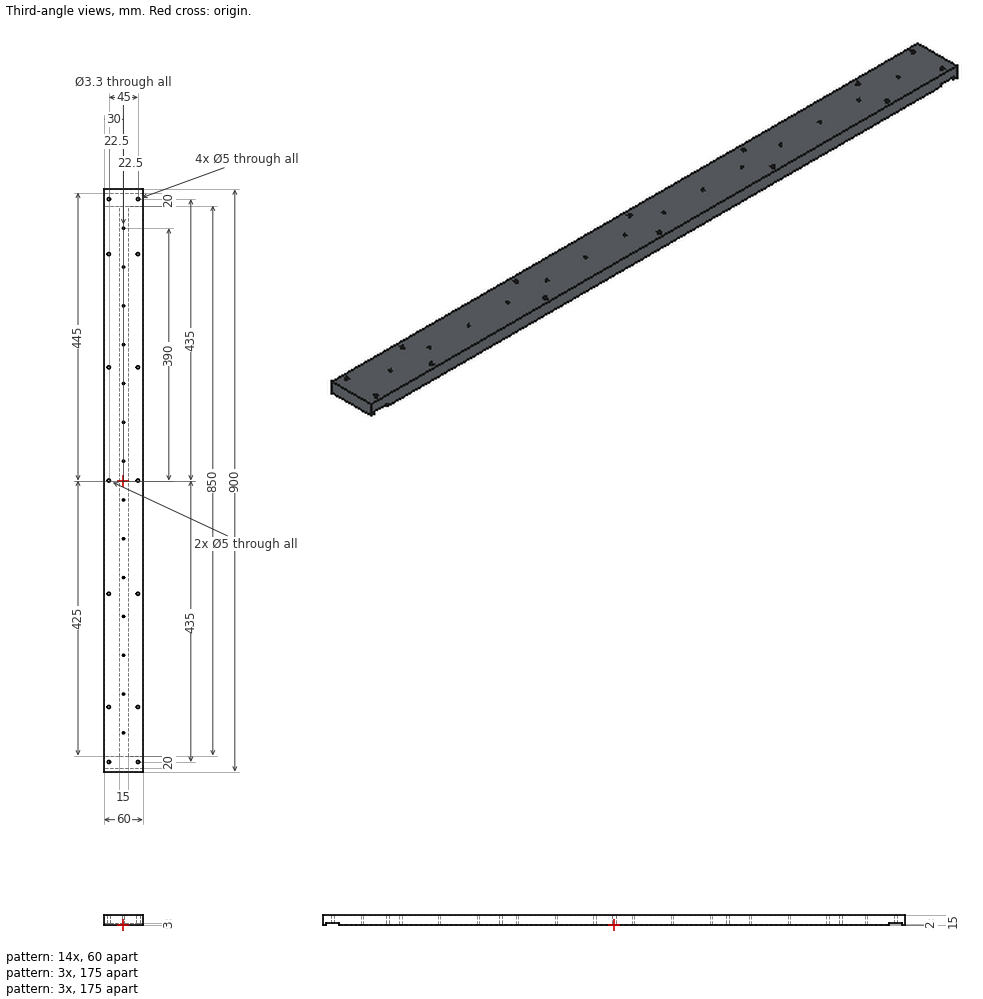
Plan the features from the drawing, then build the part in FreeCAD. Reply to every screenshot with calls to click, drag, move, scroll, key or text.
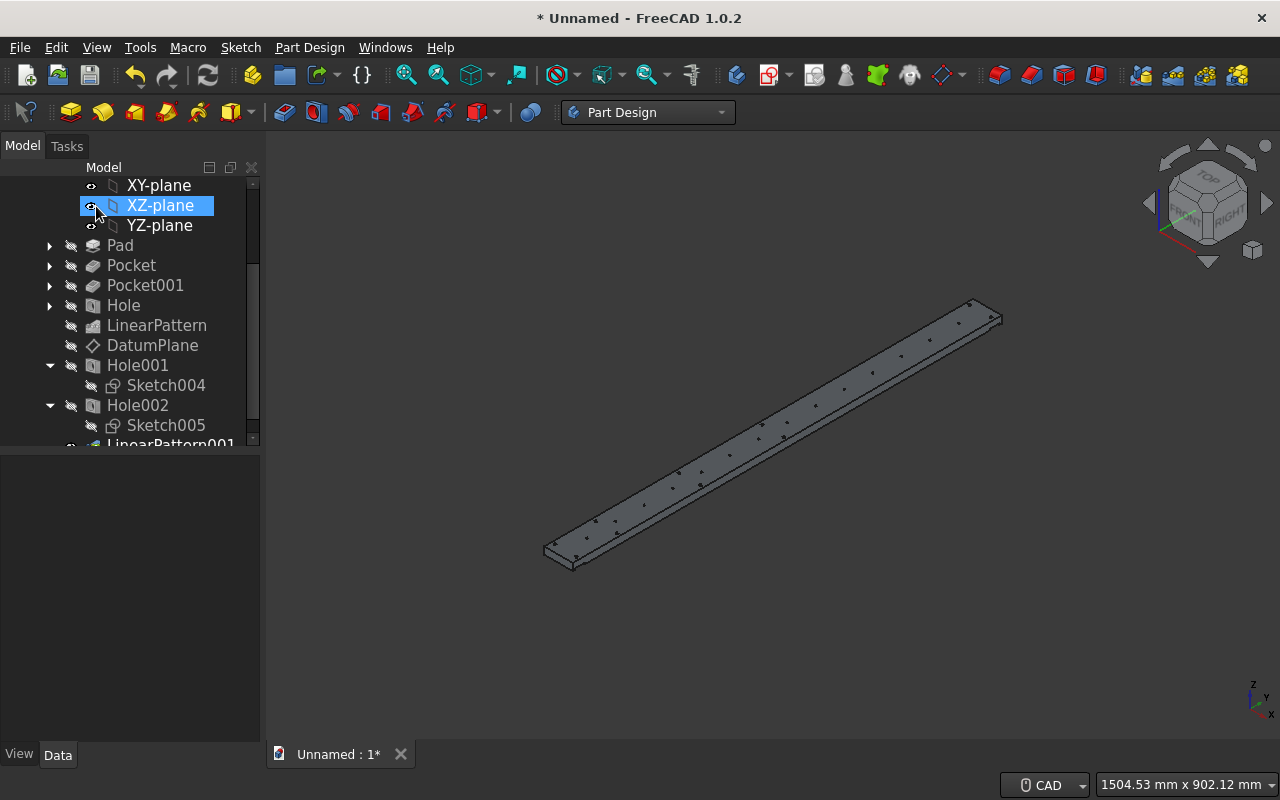
click(116, 406)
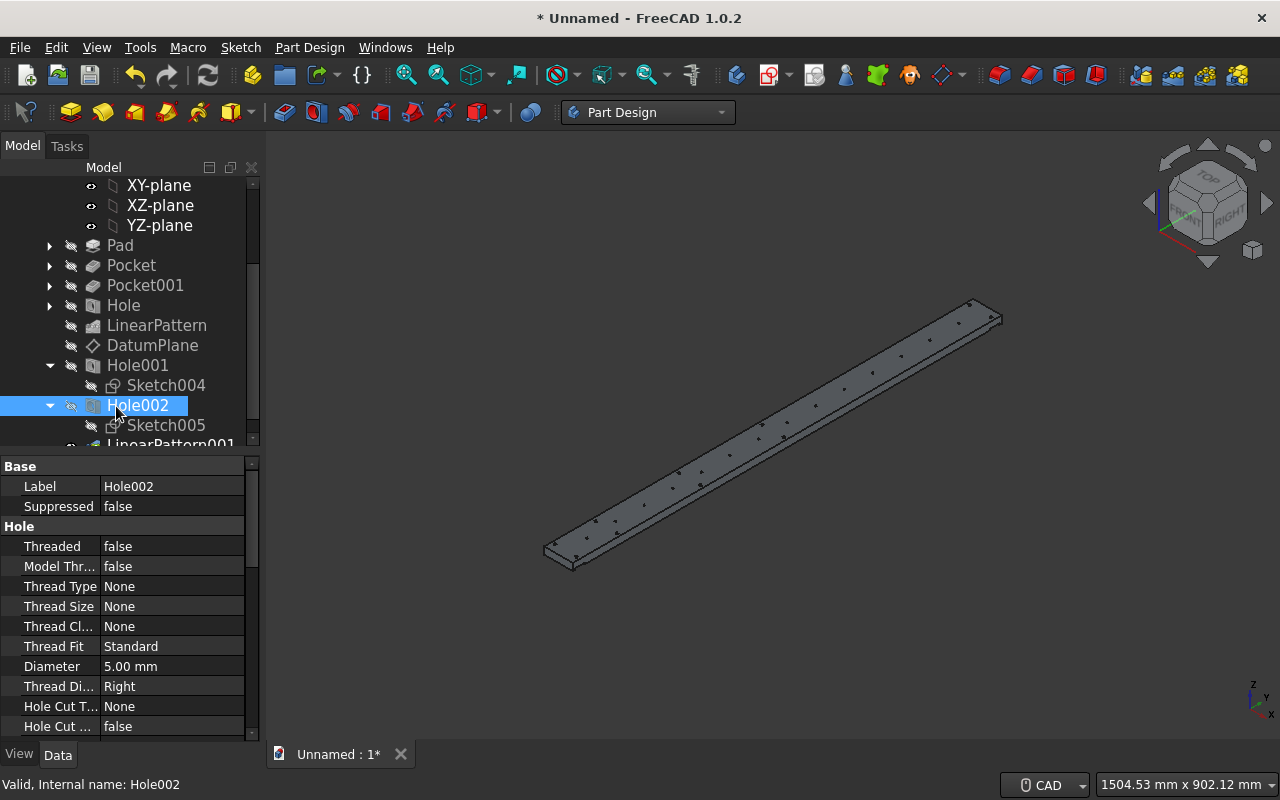
click(1174, 76)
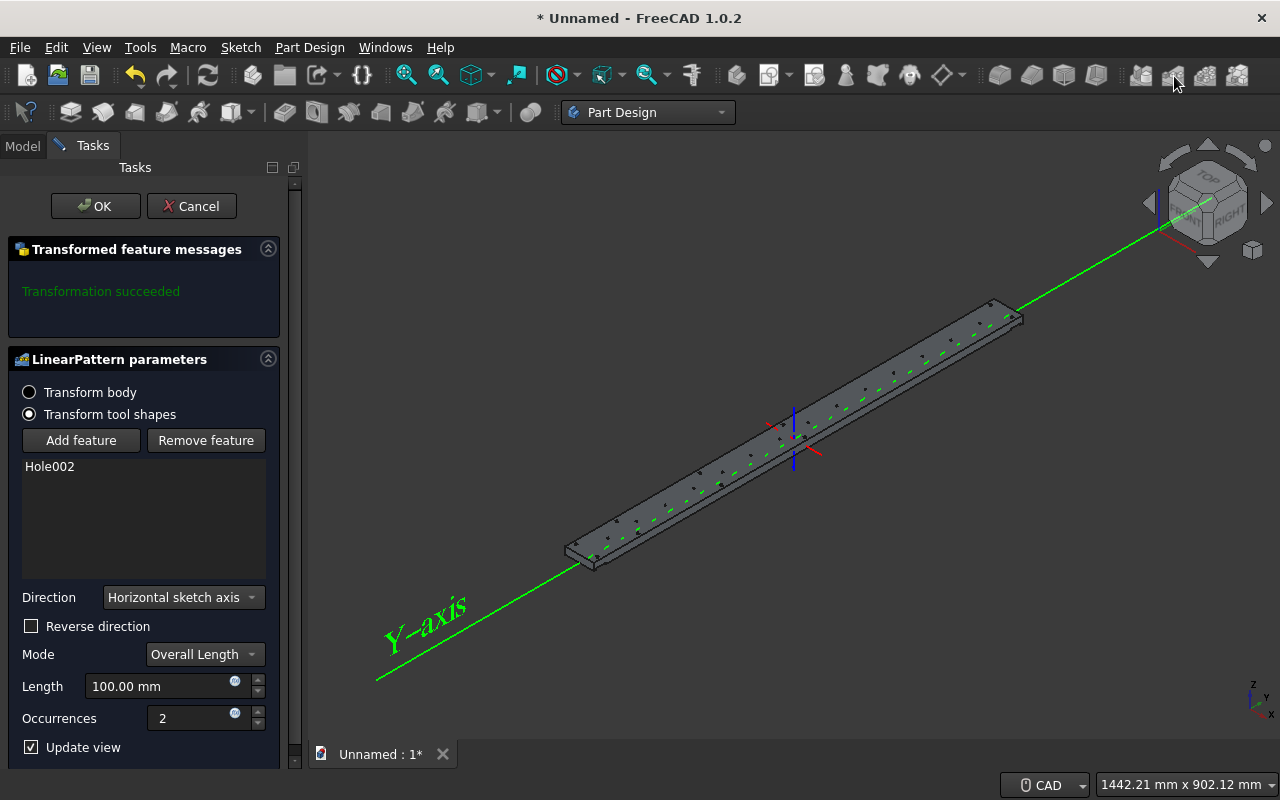
click(184, 598)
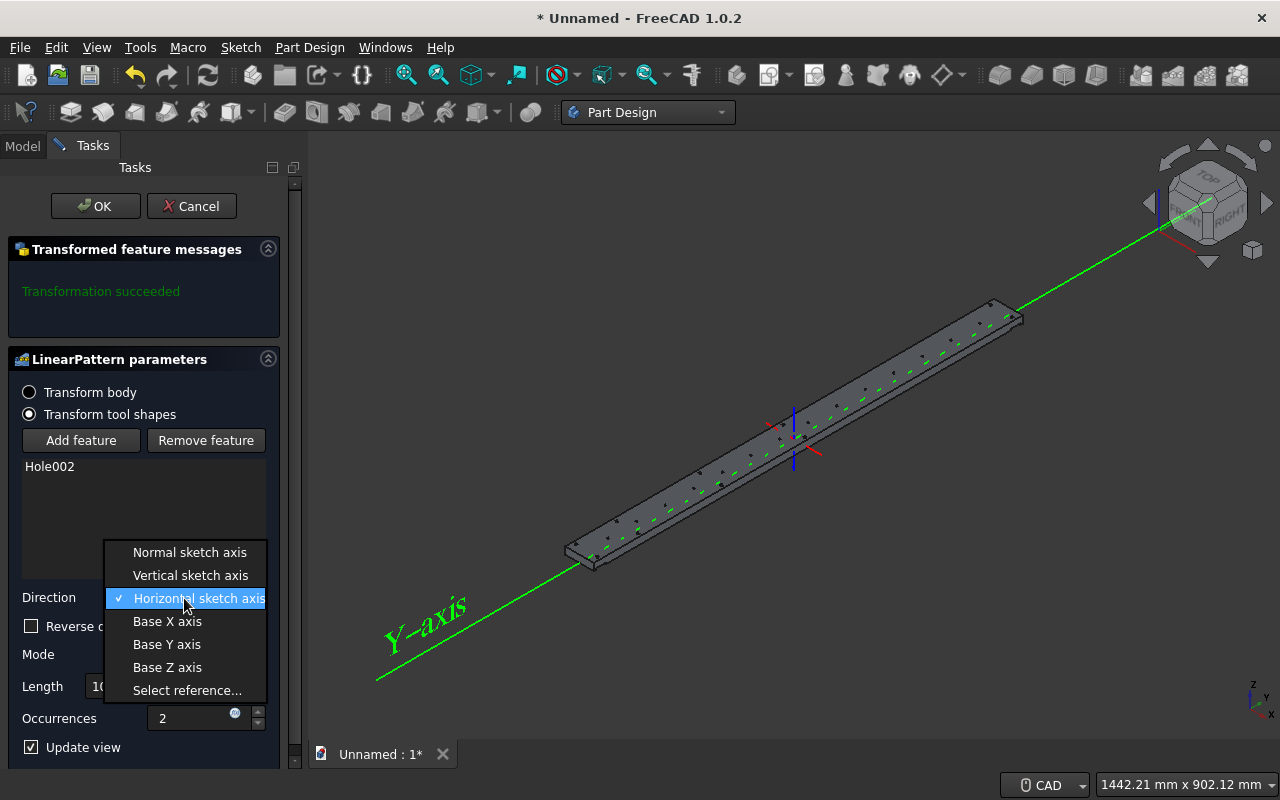
click(184, 644)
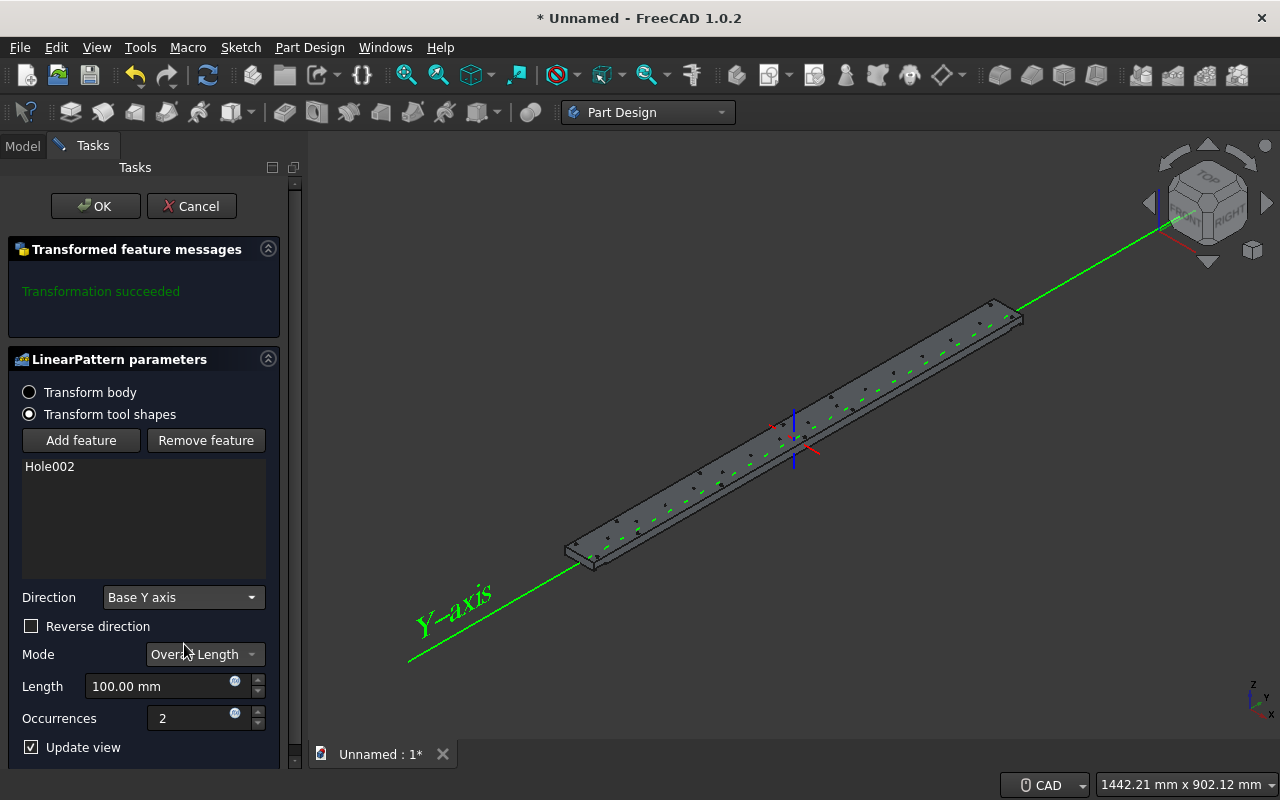
click(206, 654)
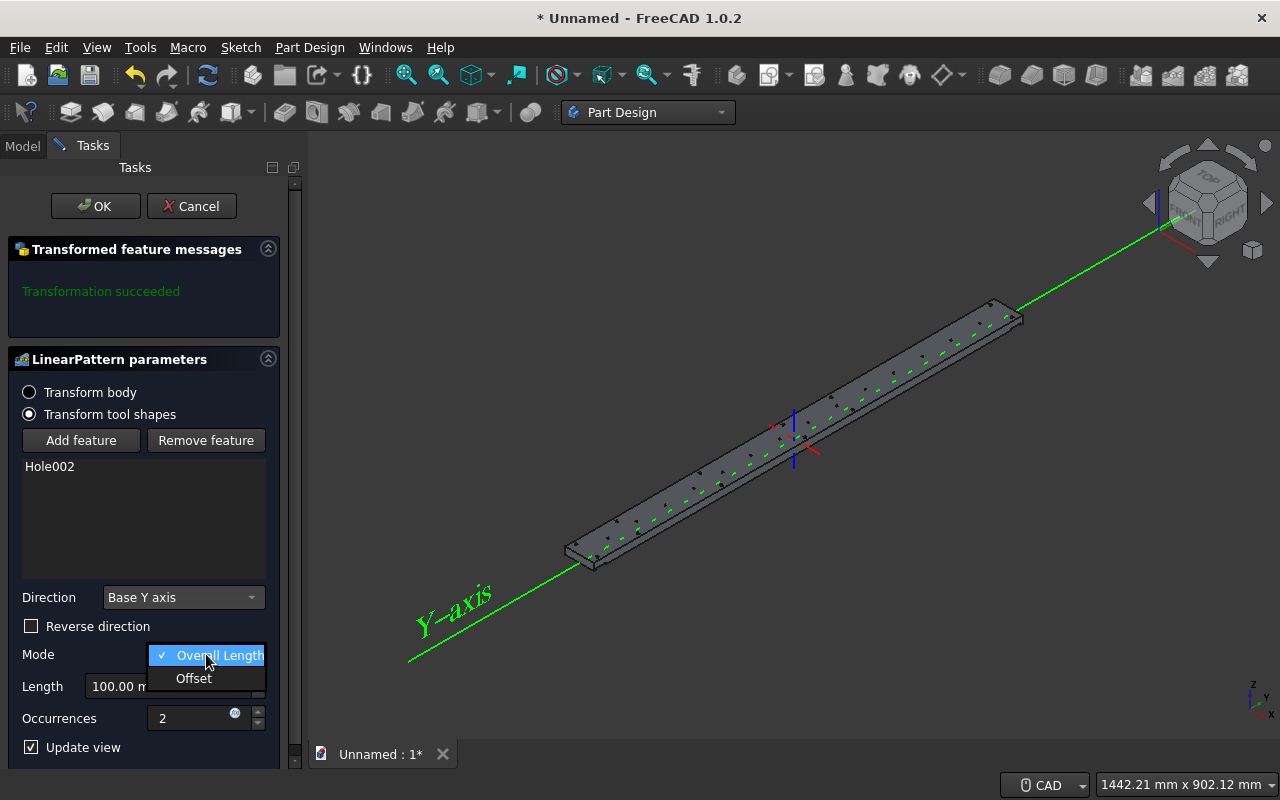
click(206, 678)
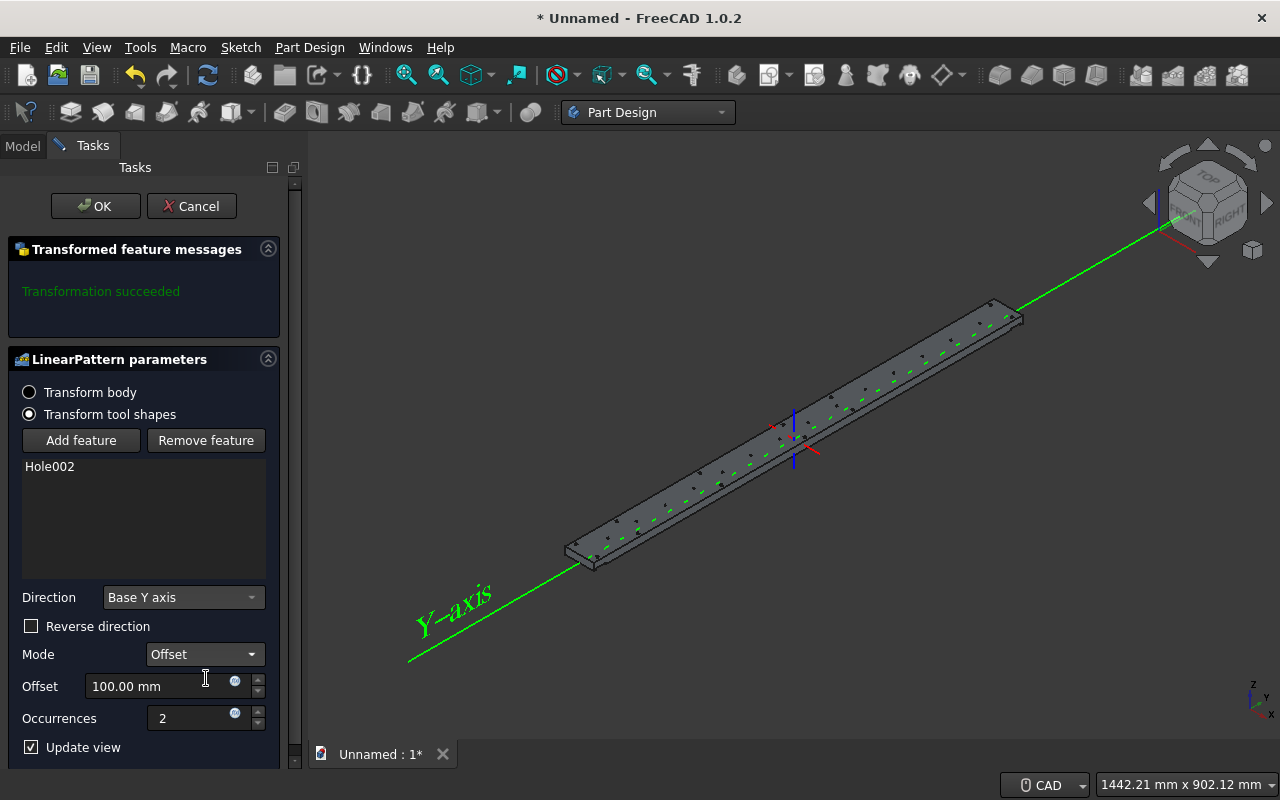
triple_click(168, 686)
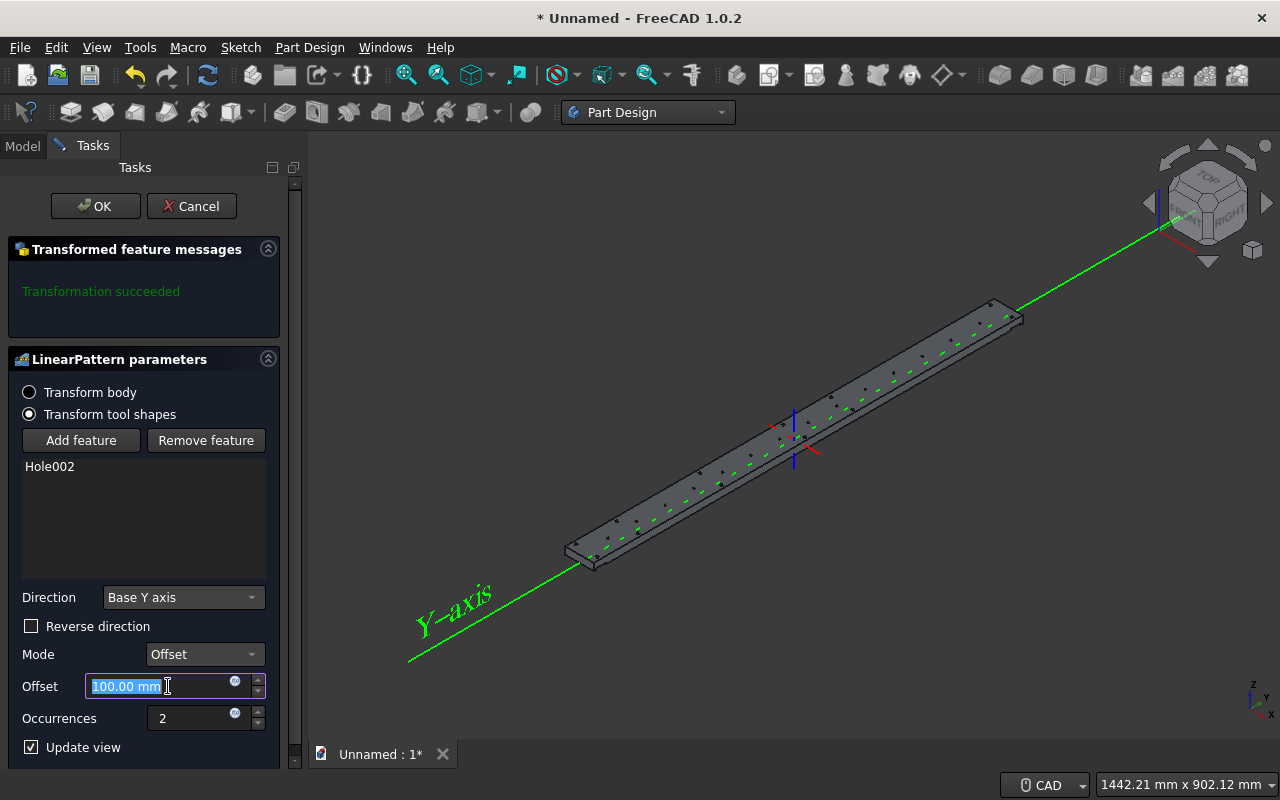
text(175)
key(Tab)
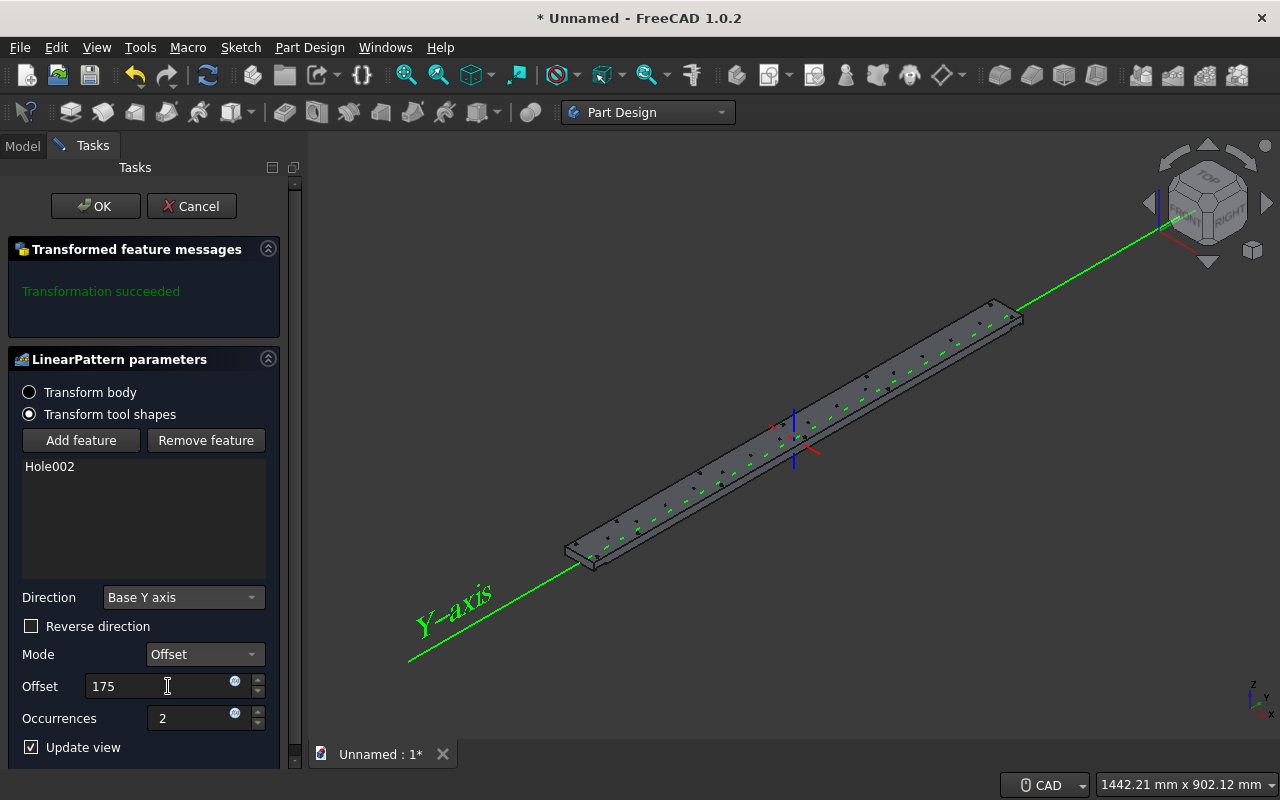
triple_click(198, 718)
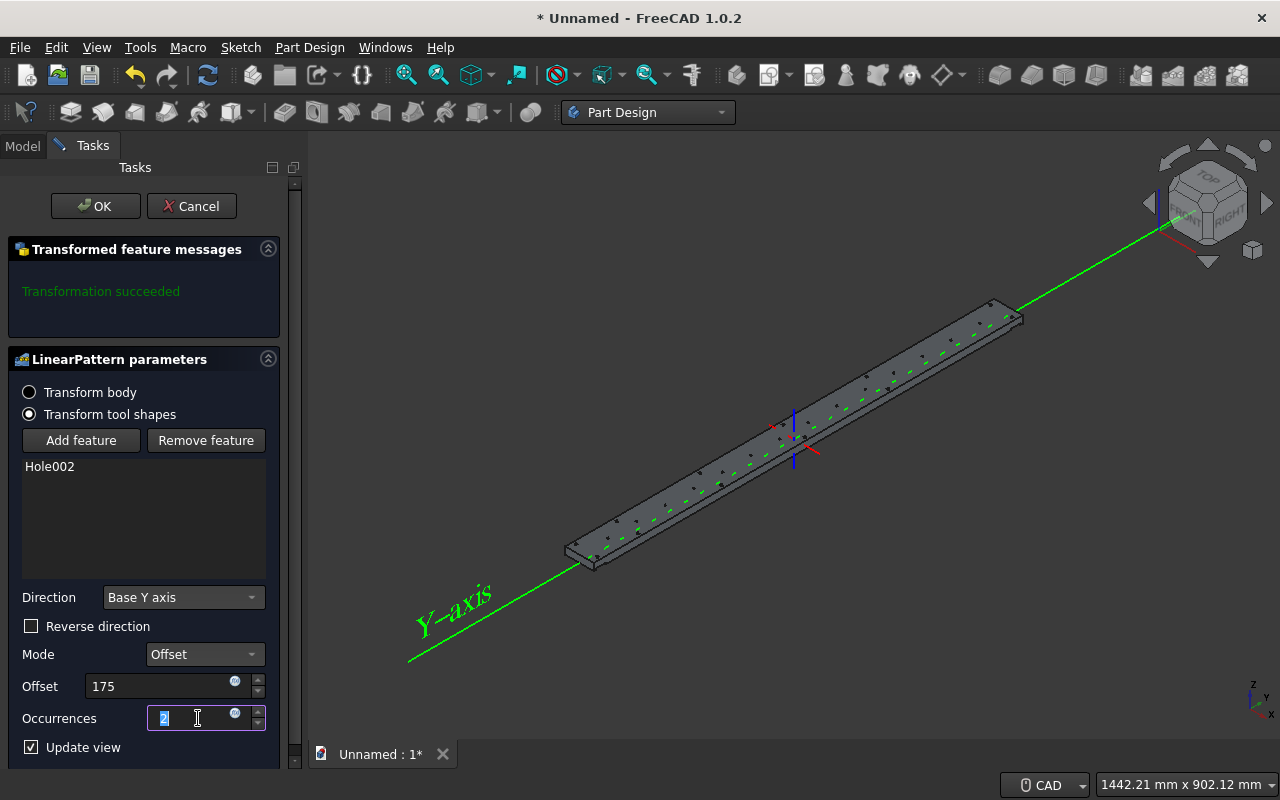
text(3)
key(Tab)